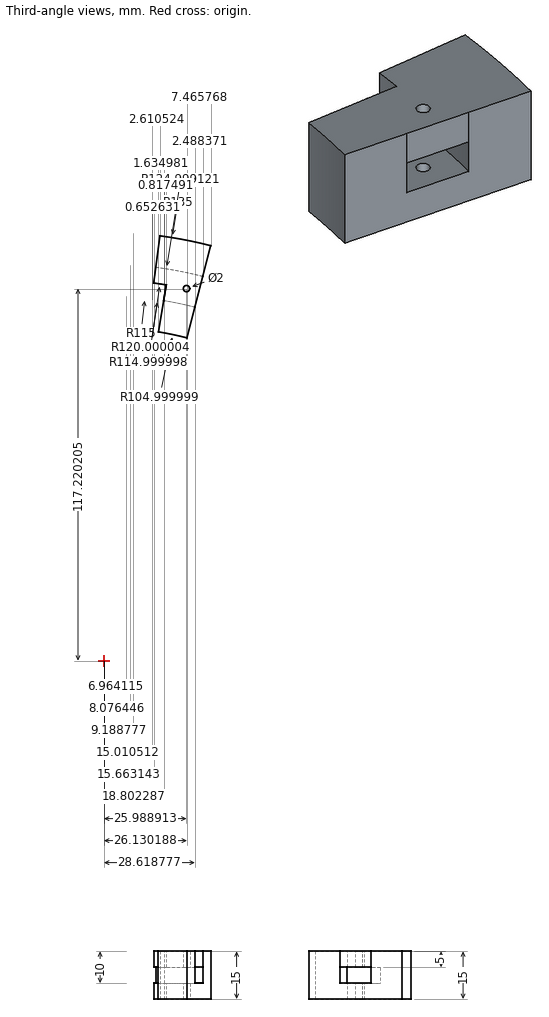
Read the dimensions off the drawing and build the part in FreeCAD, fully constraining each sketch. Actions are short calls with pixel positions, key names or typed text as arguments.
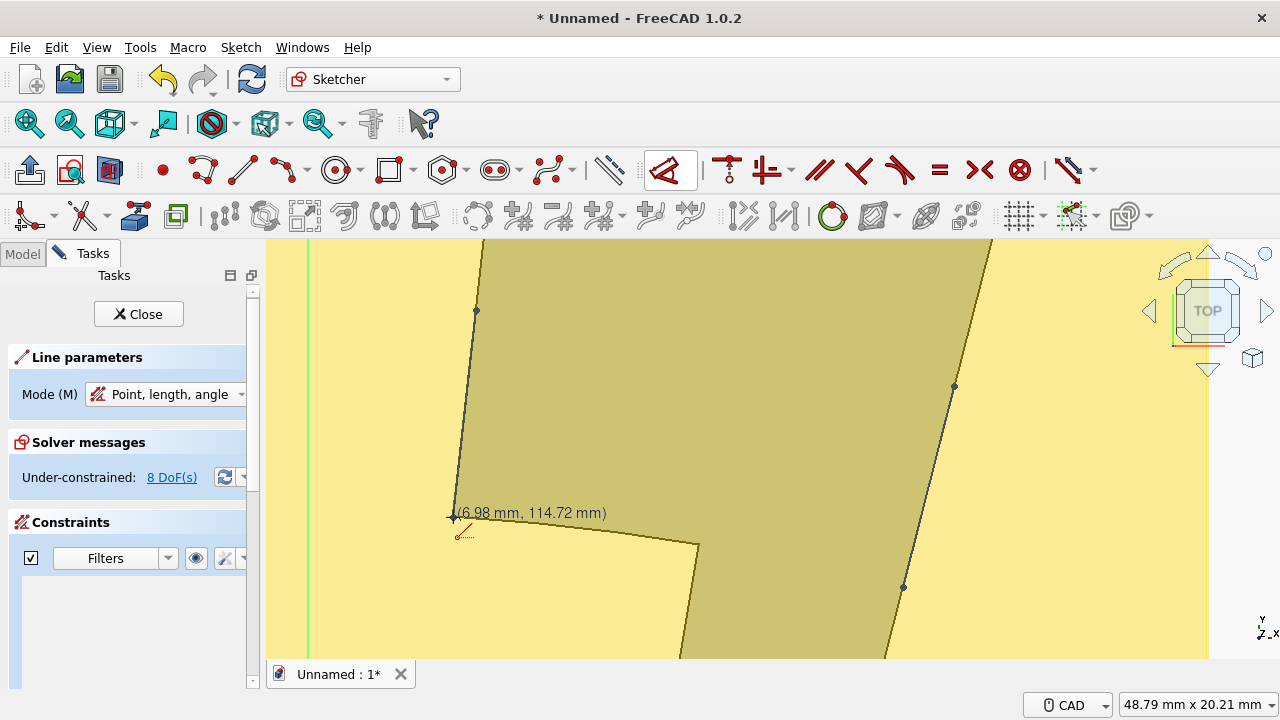
click(284, 170)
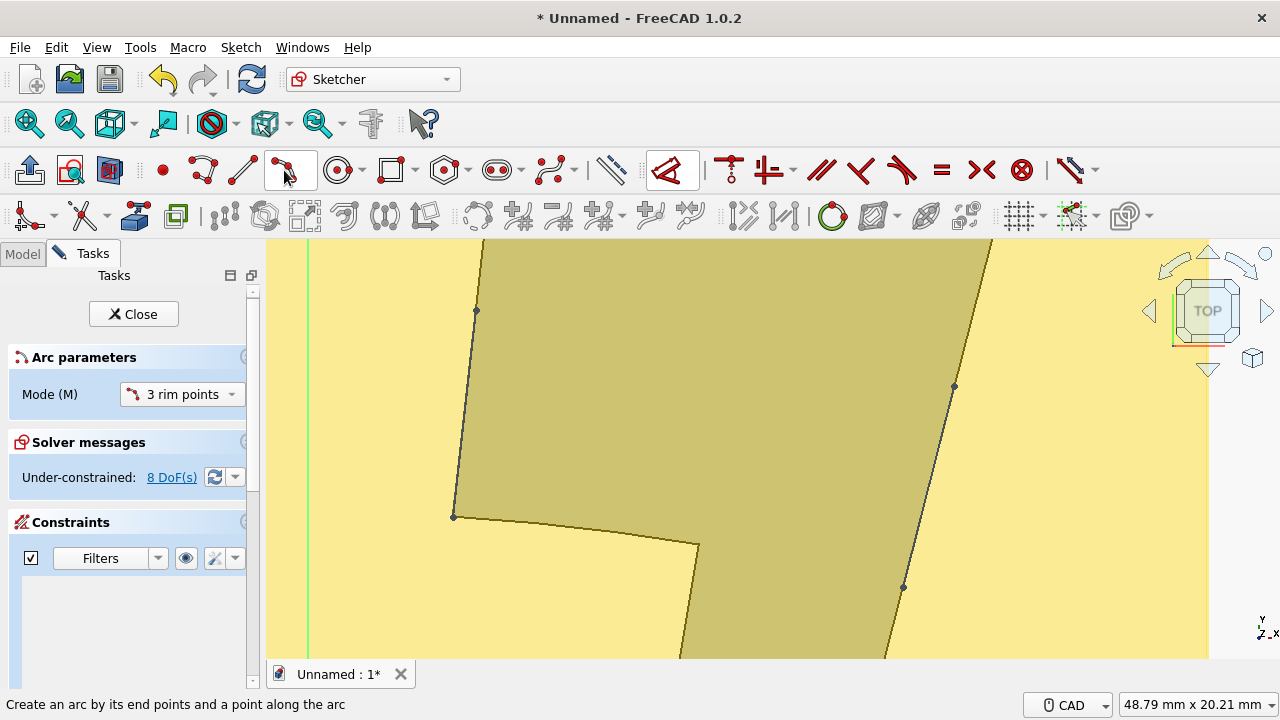
click(954, 387)
click(476, 311)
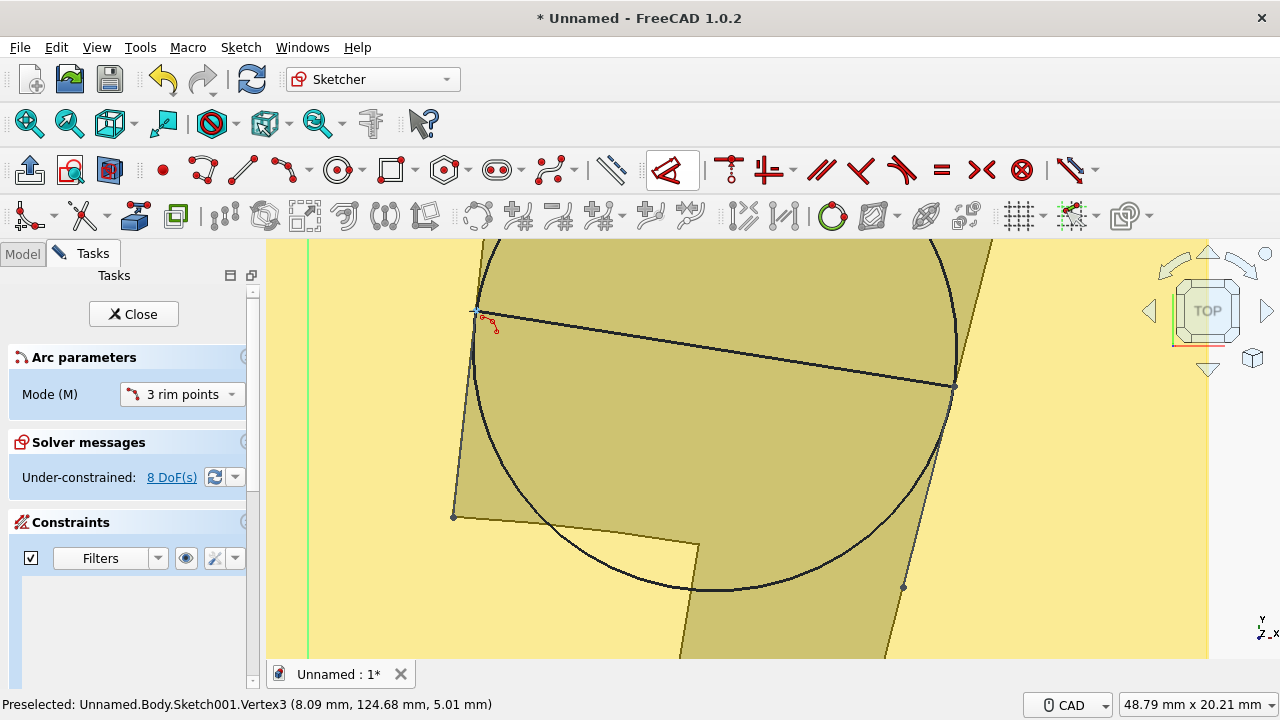
scroll(717, 337, up, 2)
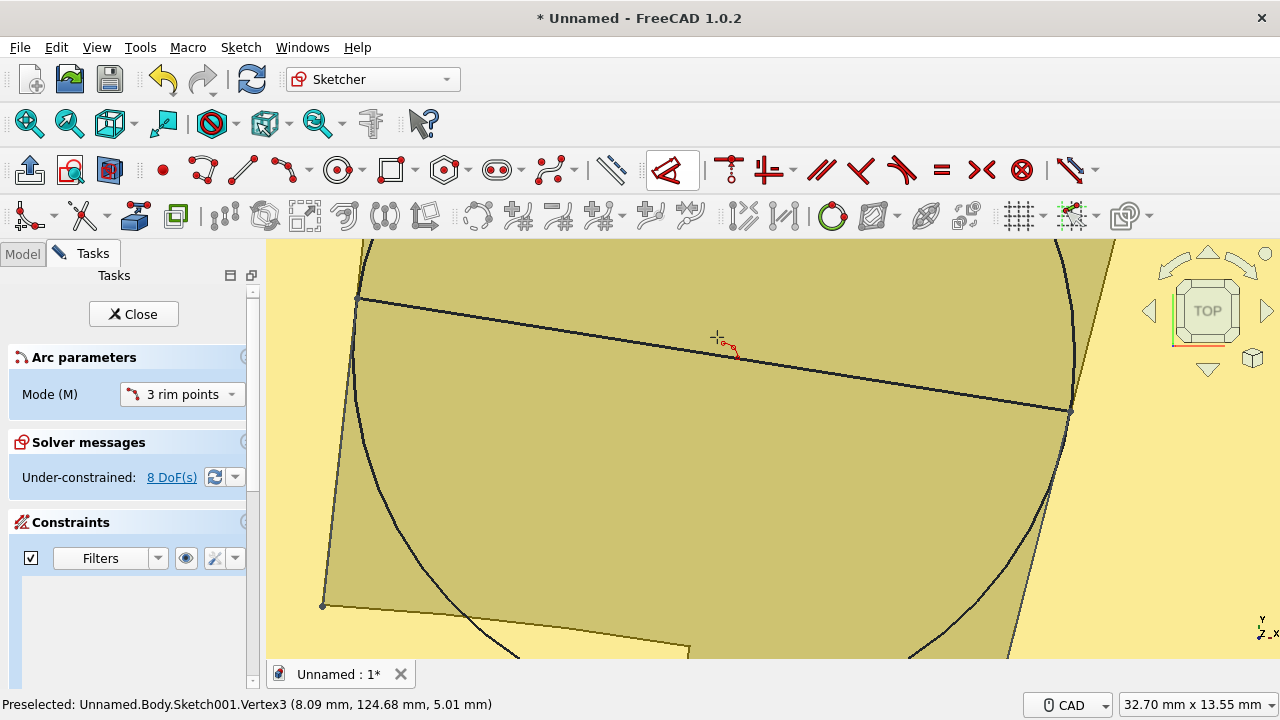
click(717, 337)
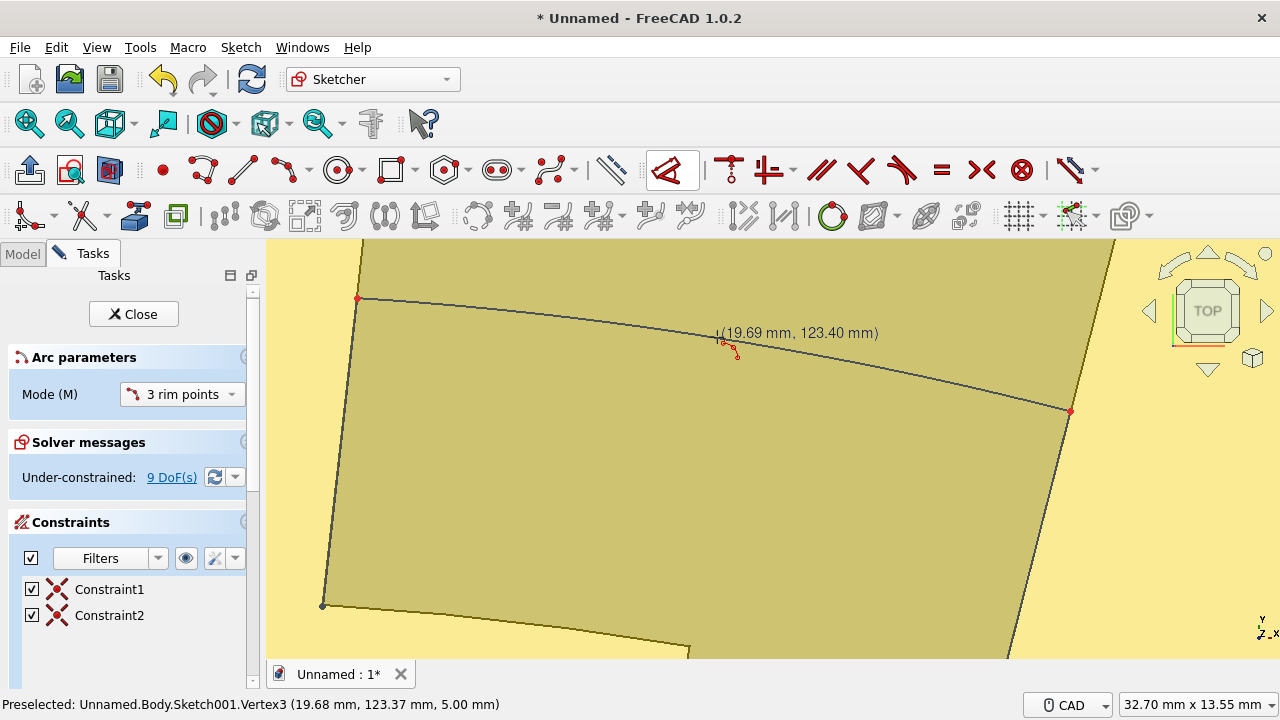
click(323, 607)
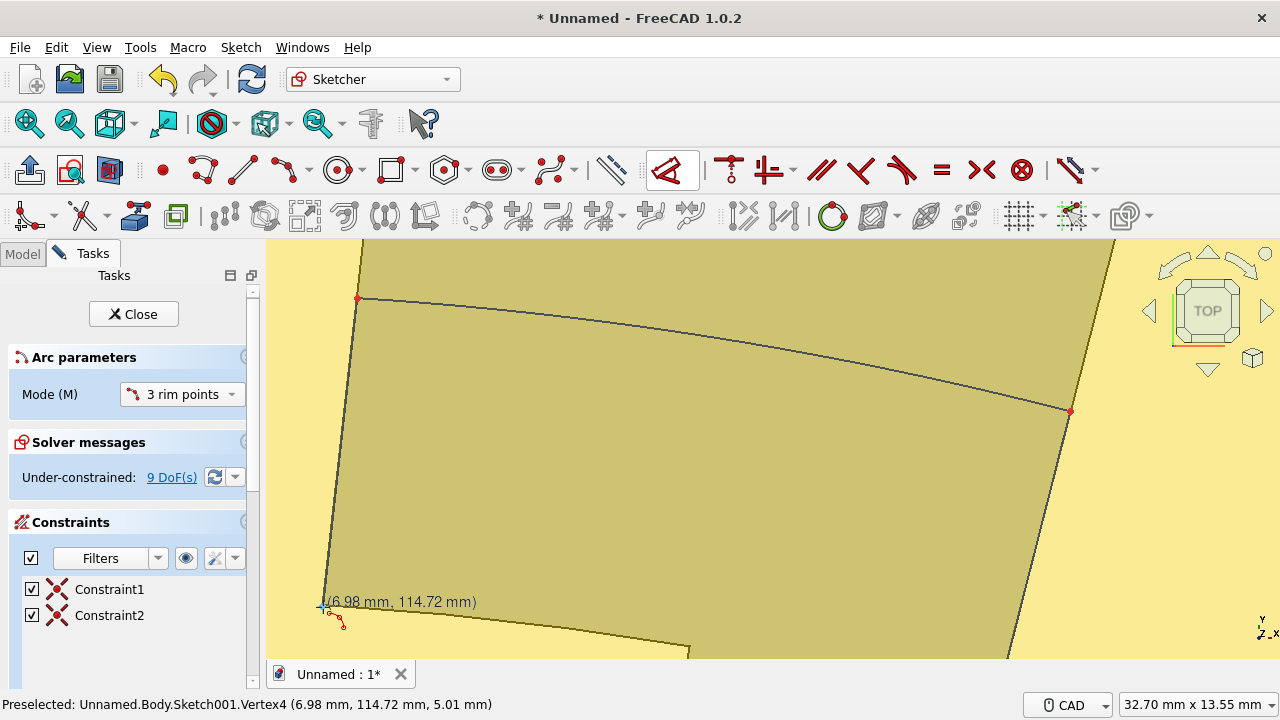
scroll(720, 338, down, 2)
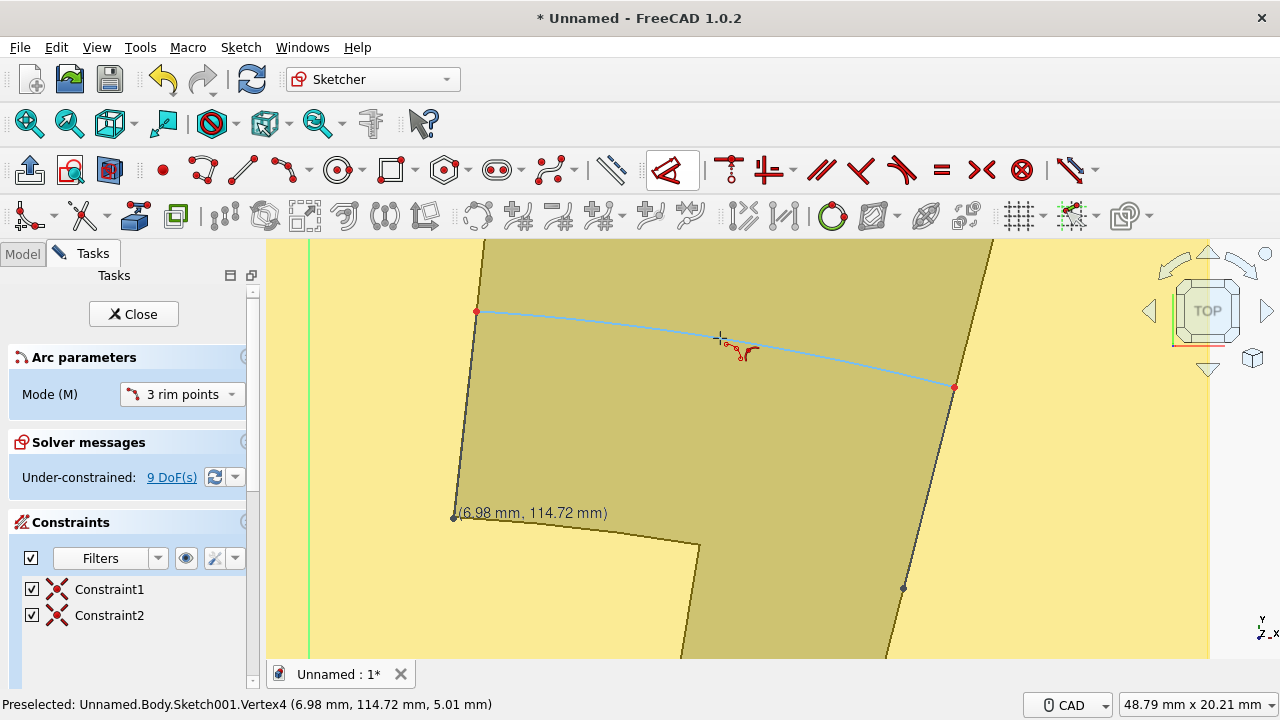
click(904, 588)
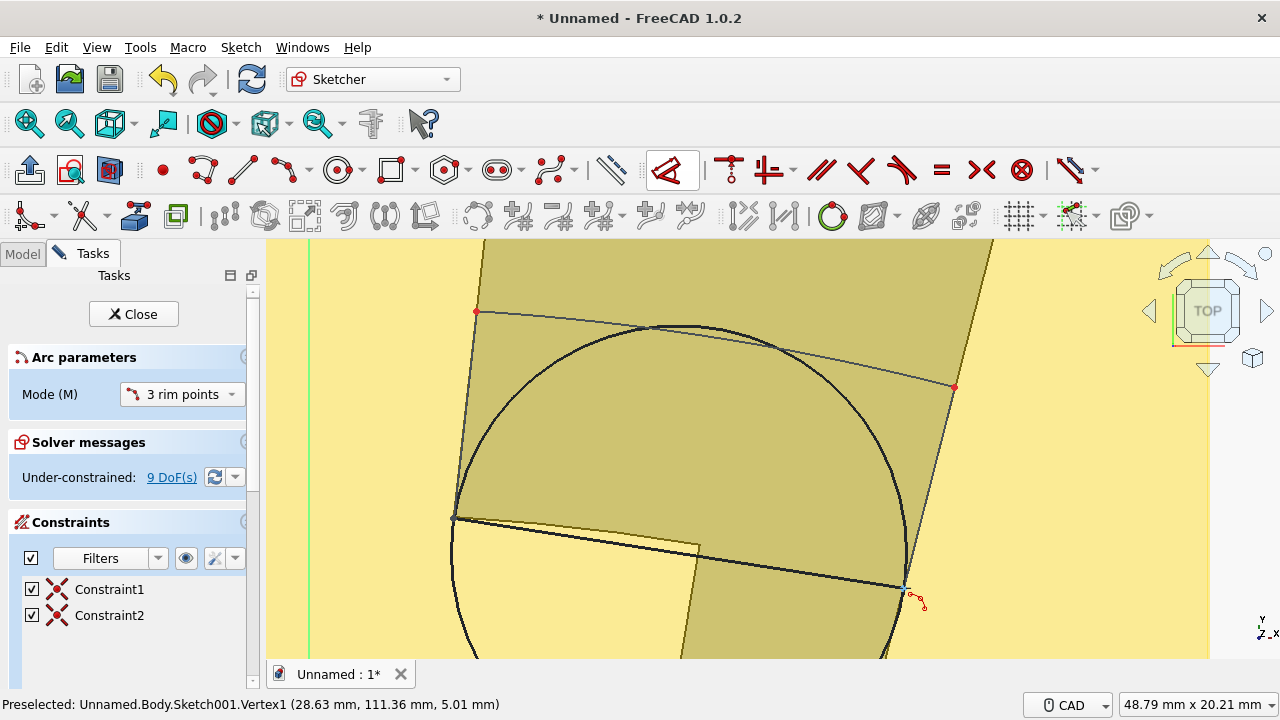
scroll(680, 542, up, 2)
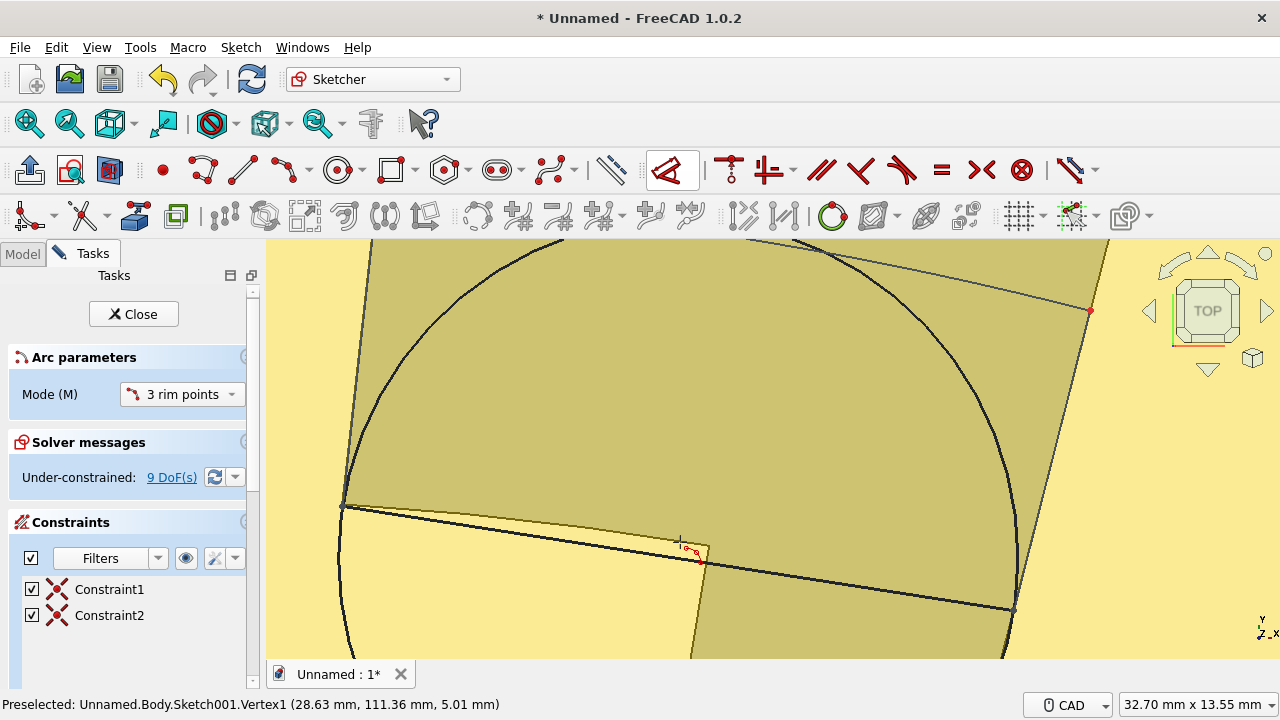
click(680, 541)
key(Escape)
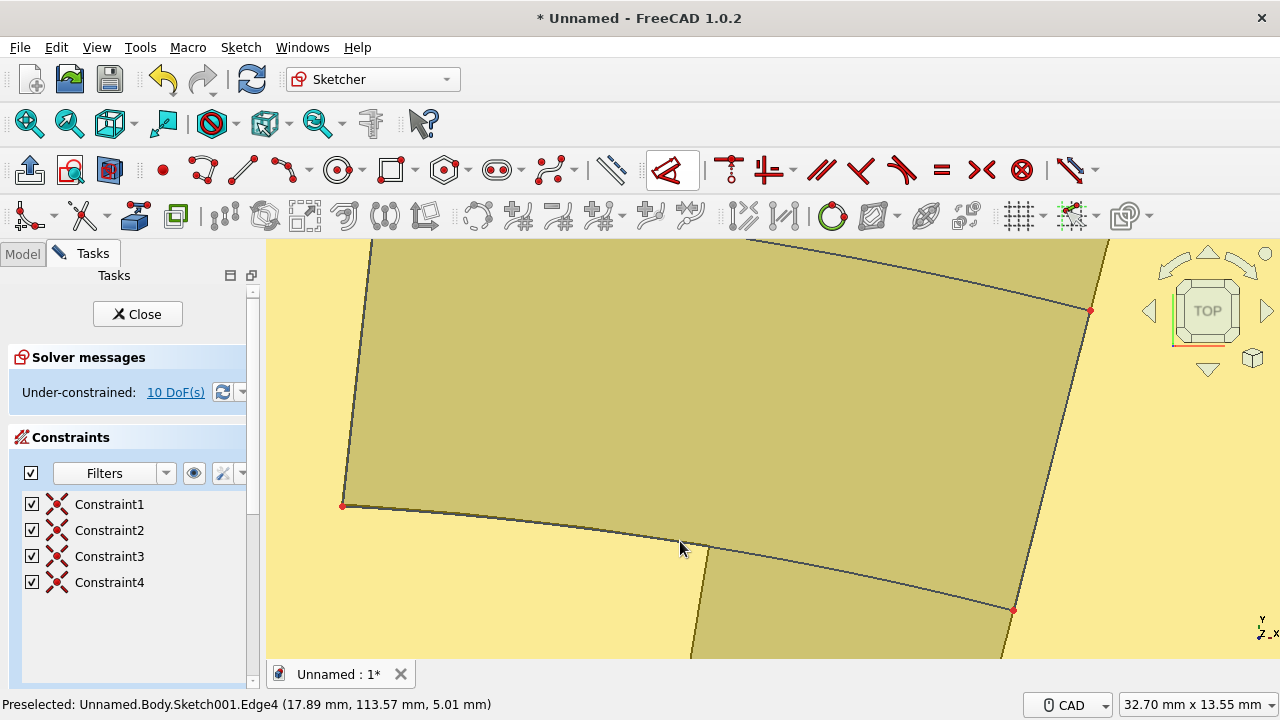
click(949, 277)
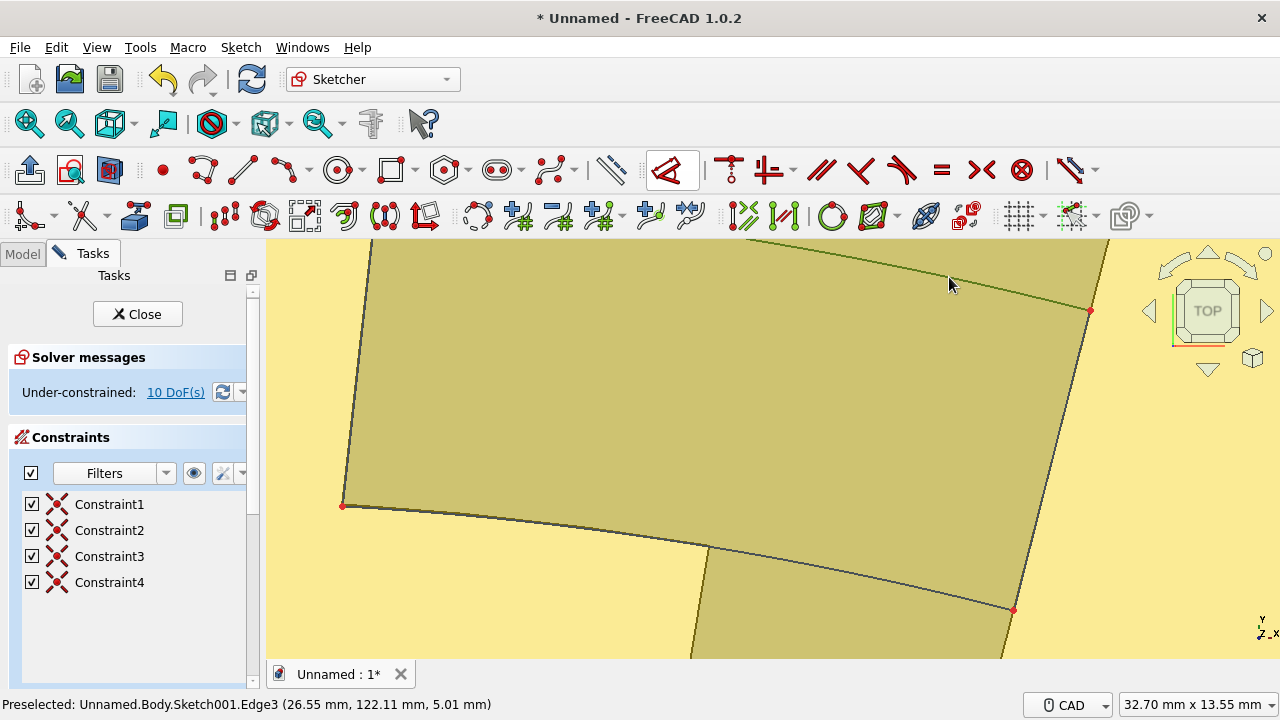
click(815, 566)